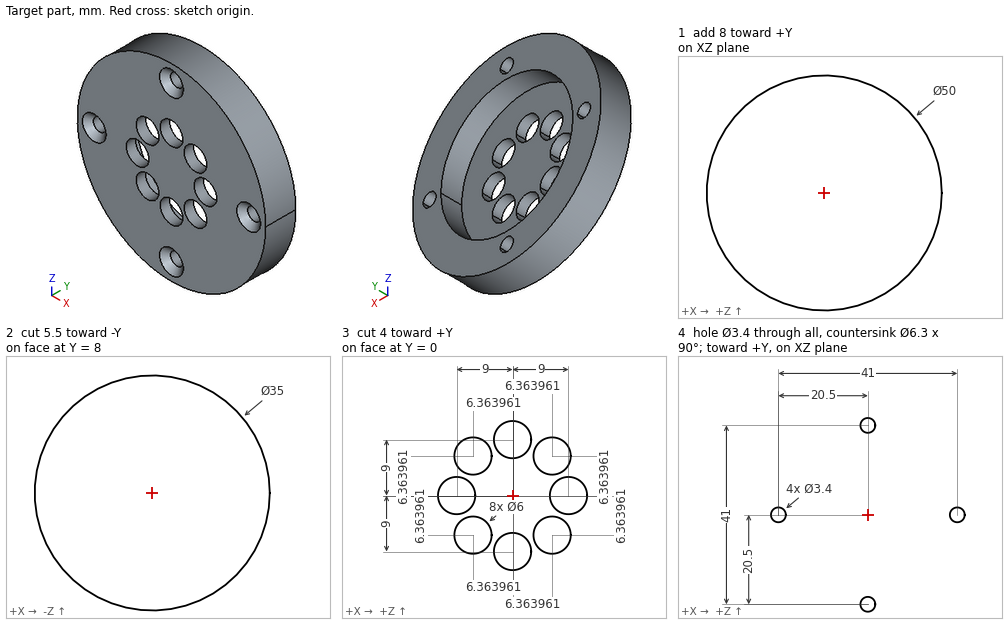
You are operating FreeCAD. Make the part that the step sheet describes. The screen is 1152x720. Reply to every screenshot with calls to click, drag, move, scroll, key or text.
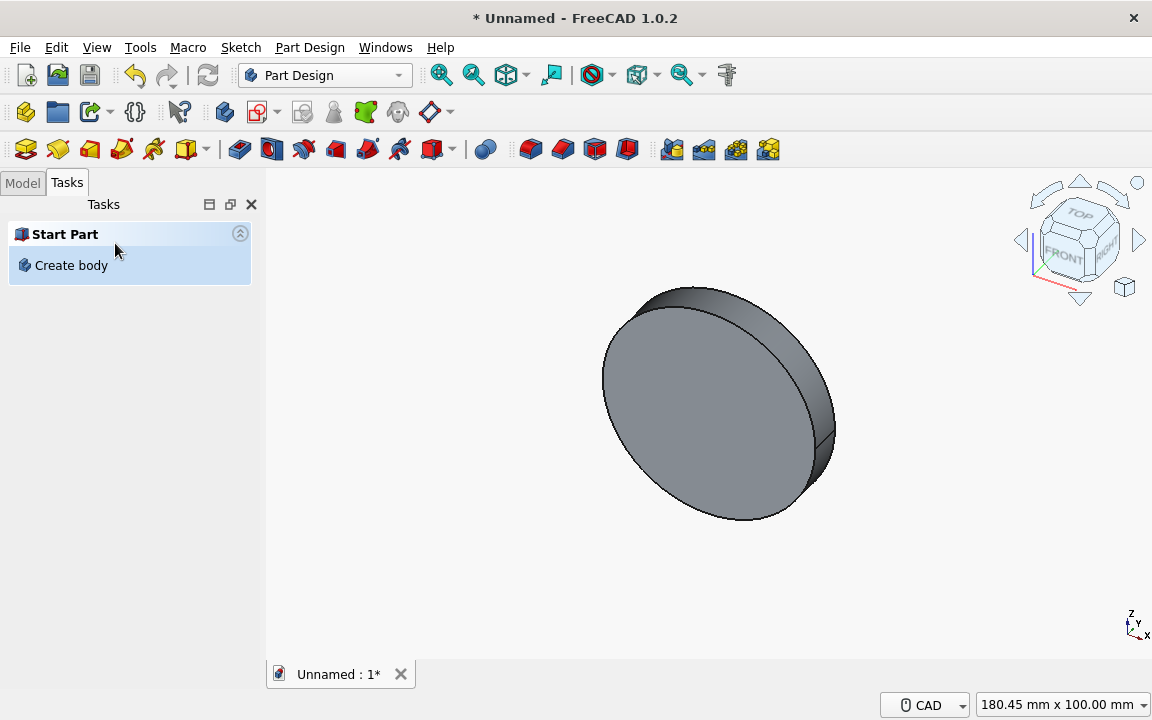
key(4)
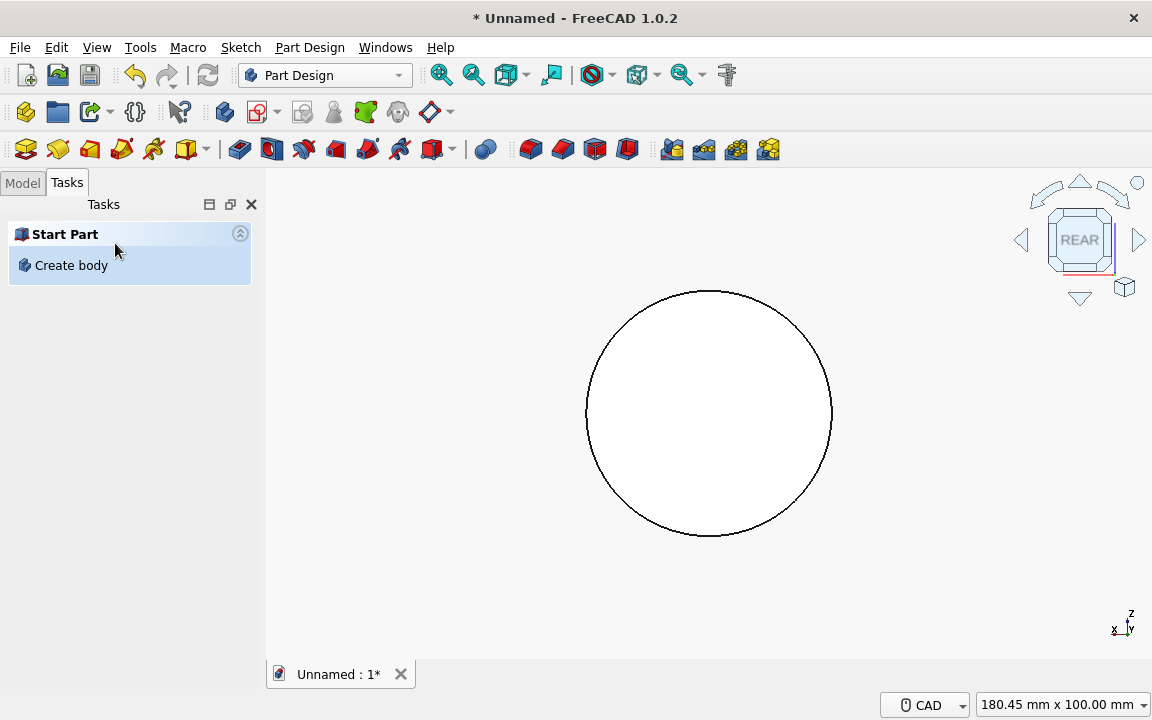
click(709, 412)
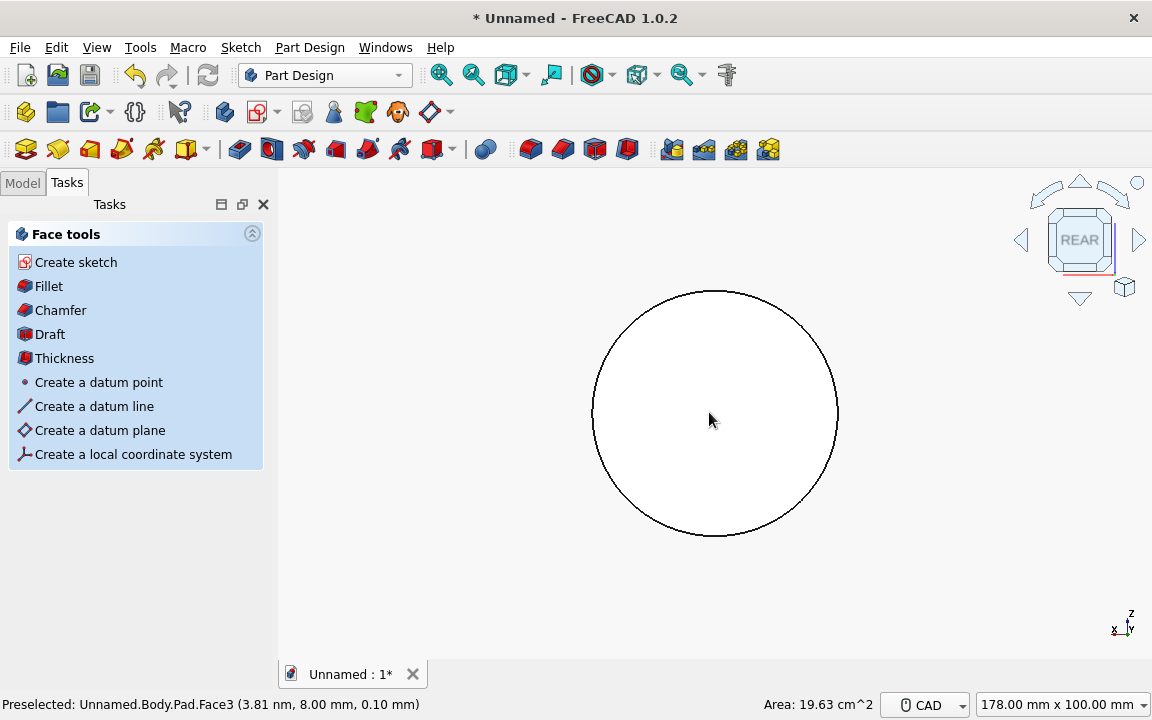
click(258, 112)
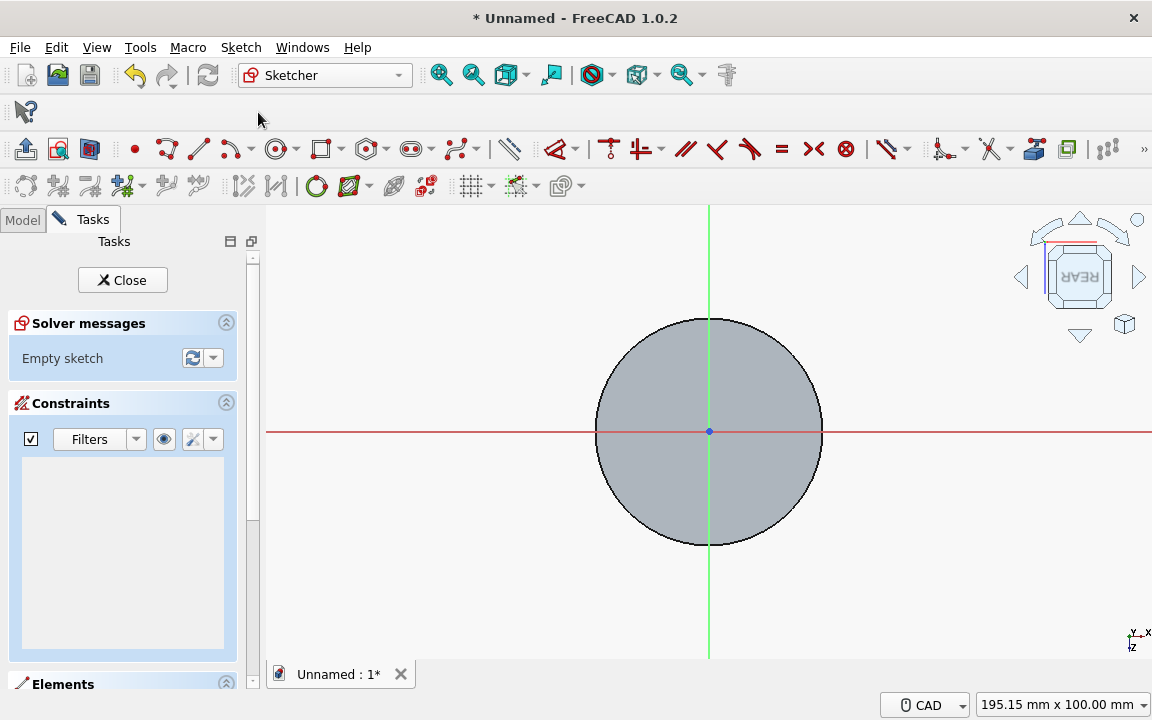
scroll(792, 432, up, 3)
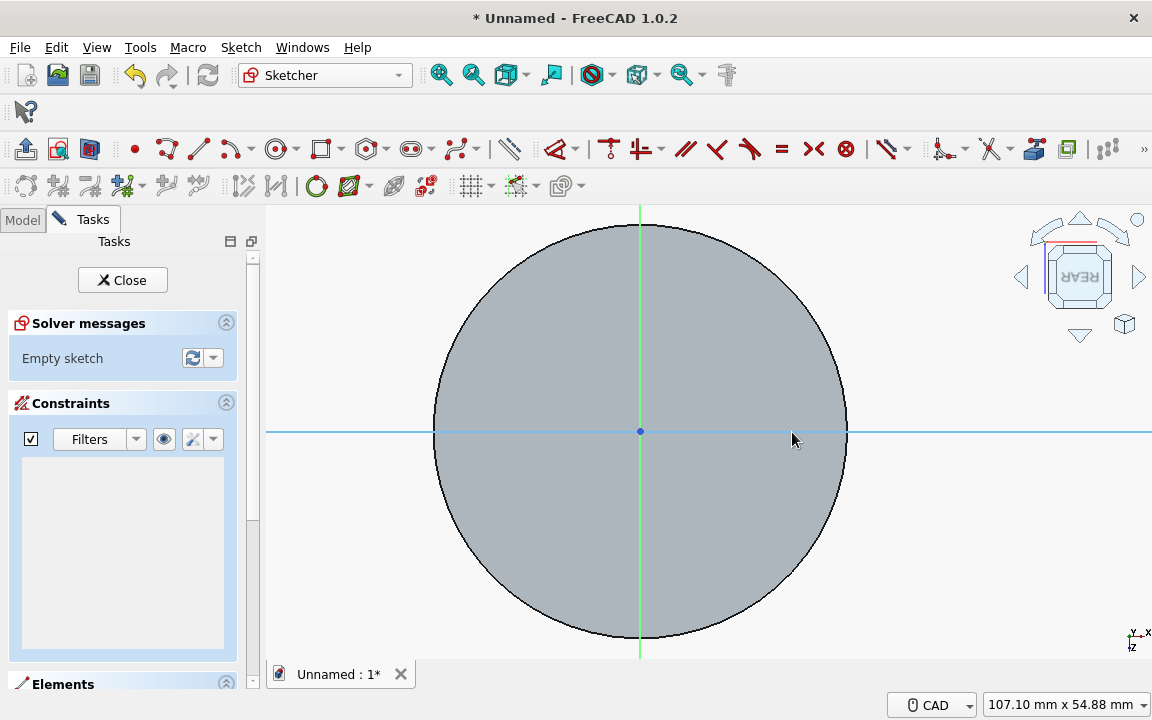
click(276, 150)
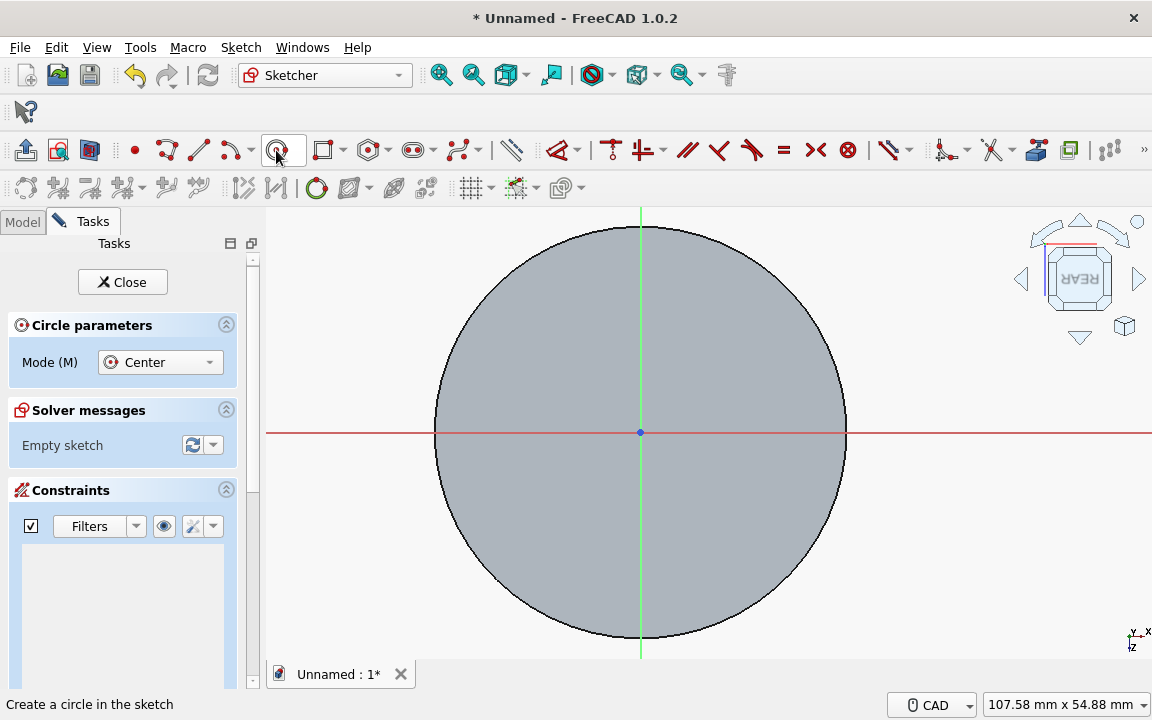
click(641, 433)
move(742, 331)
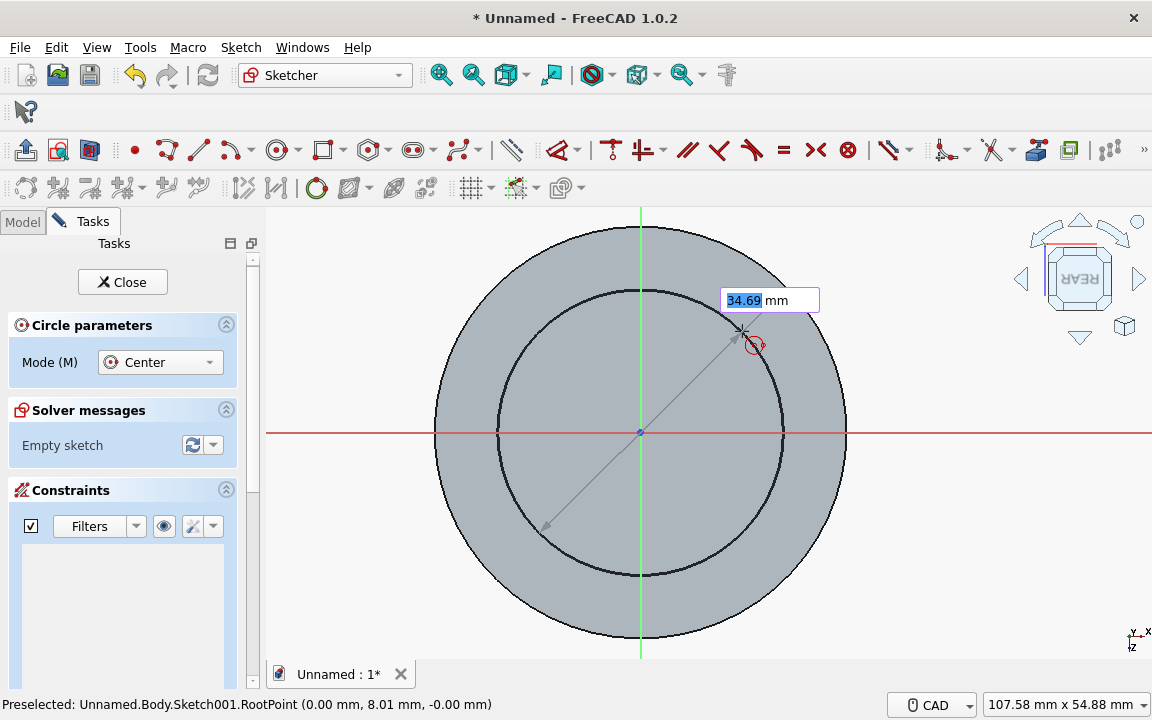
text(35)
key(Return)
key(Escape)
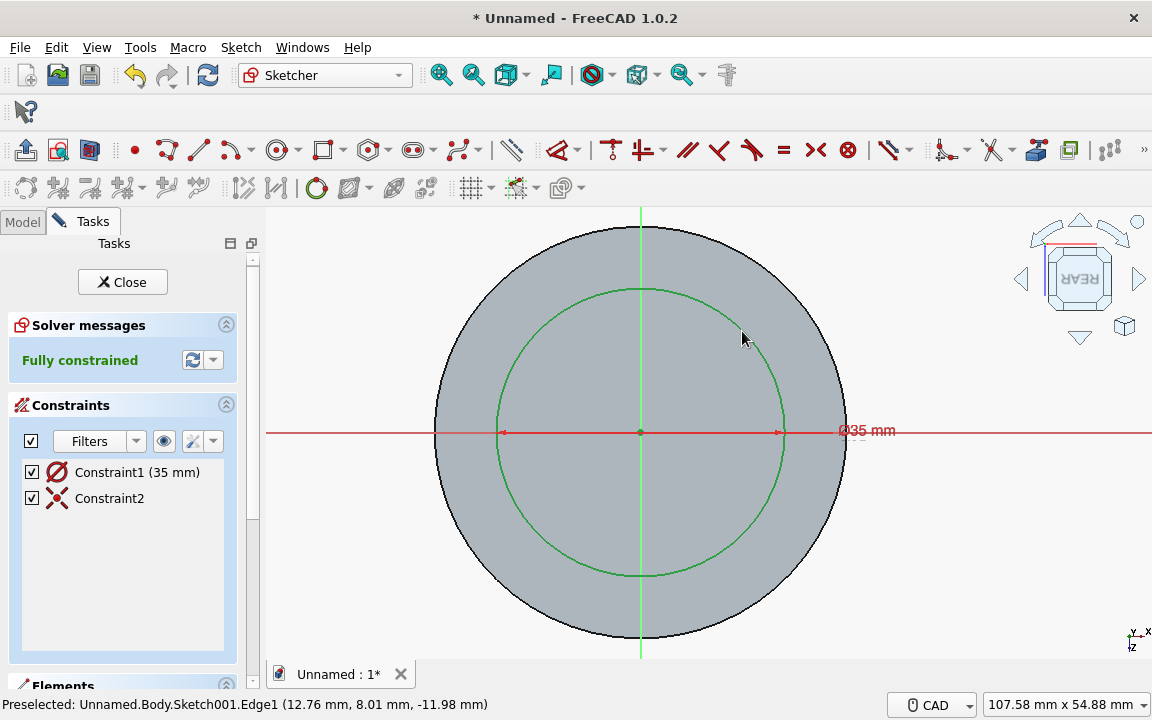
click(123, 282)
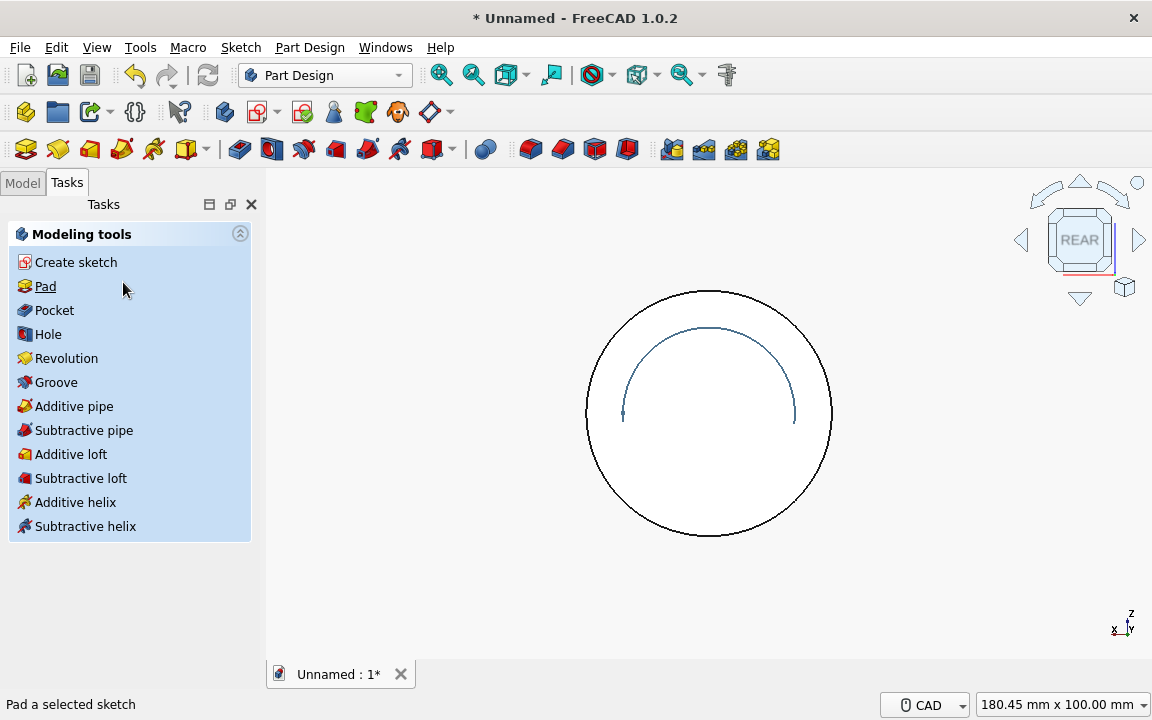
click(240, 150)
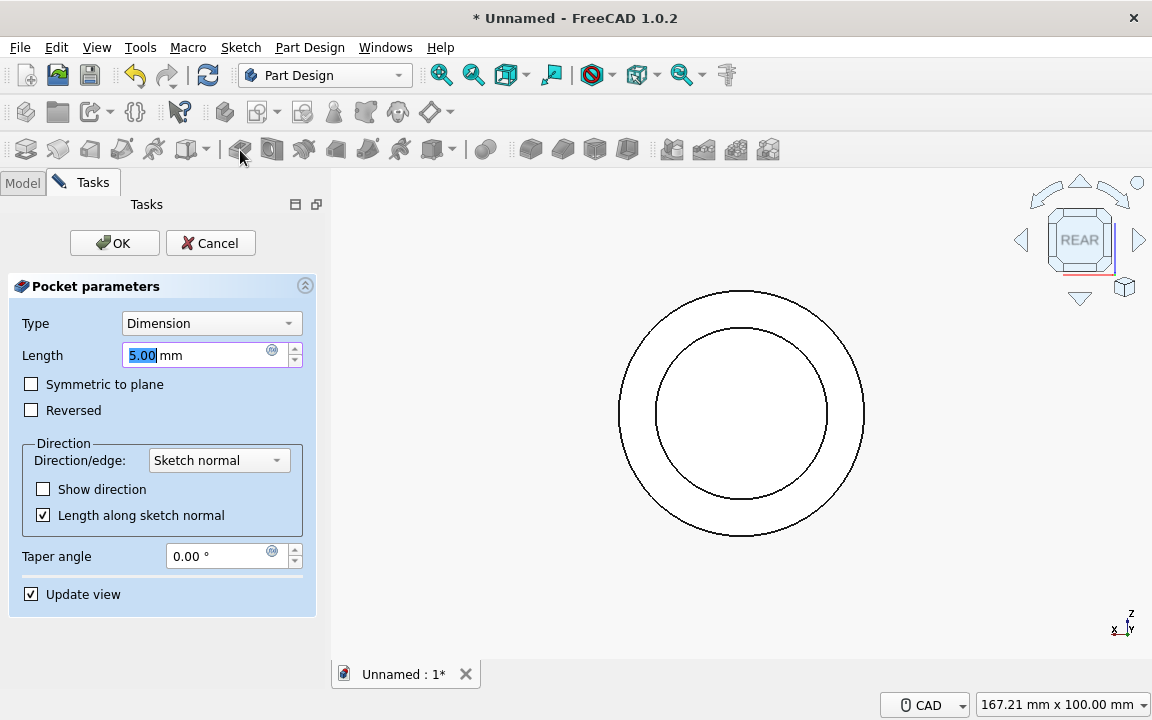
text(5.5)
key(Tab)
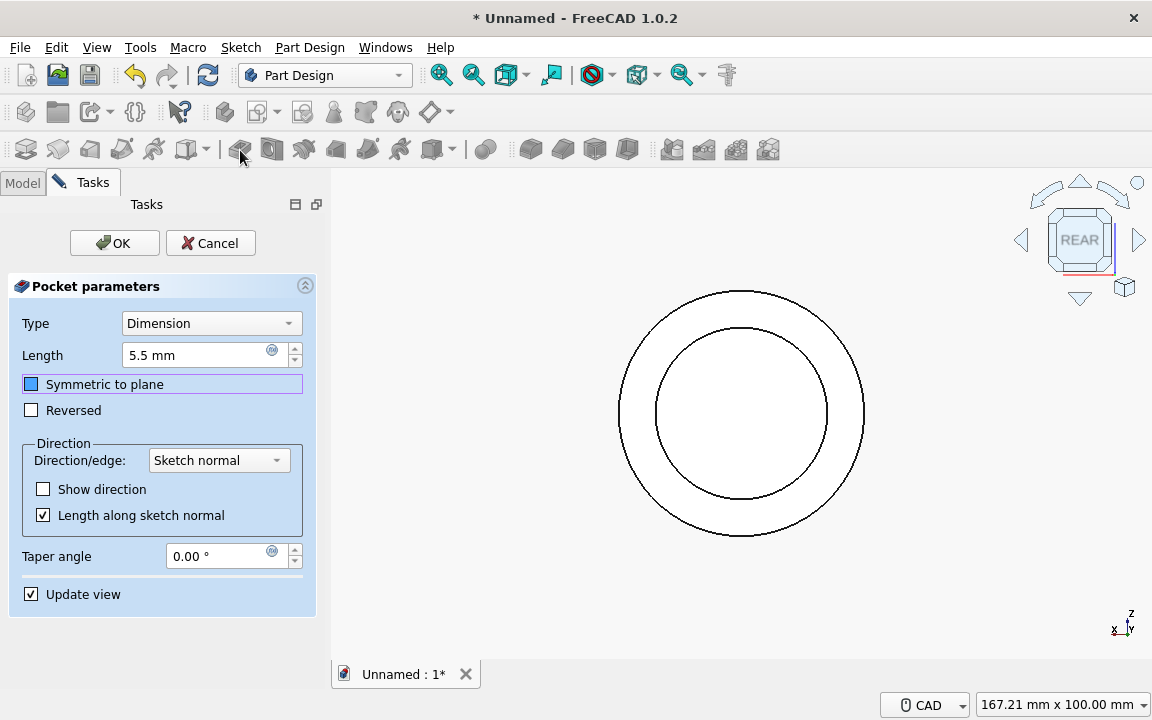
click(115, 243)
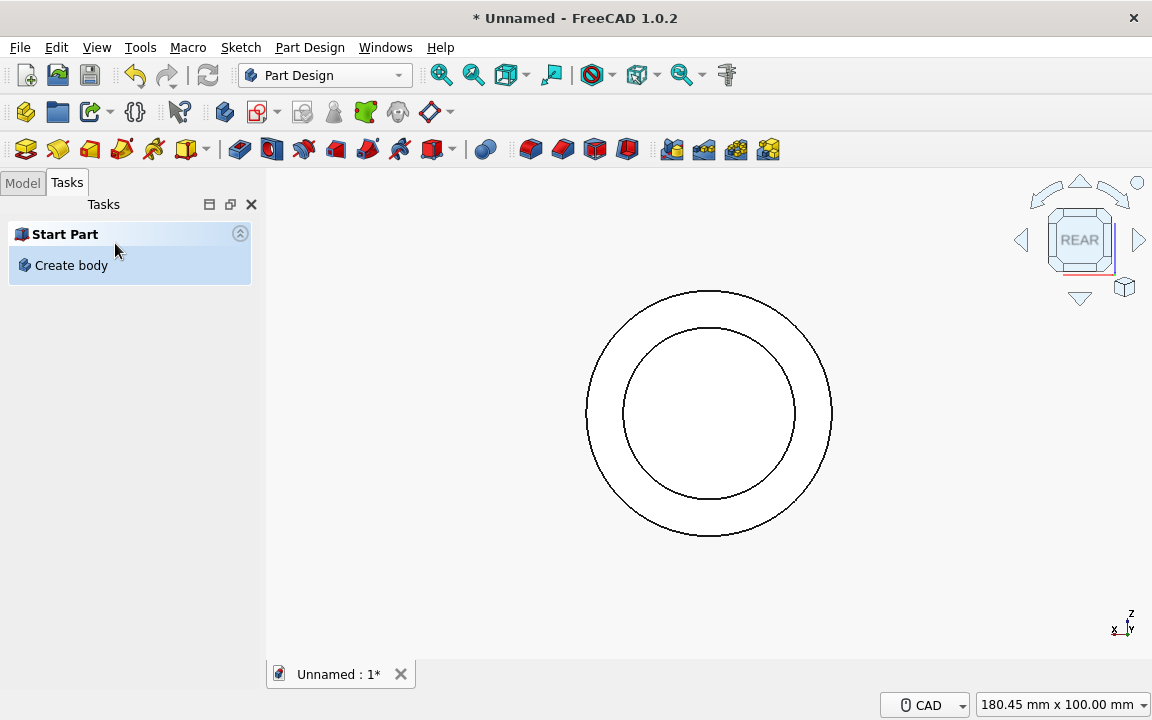
key(0)